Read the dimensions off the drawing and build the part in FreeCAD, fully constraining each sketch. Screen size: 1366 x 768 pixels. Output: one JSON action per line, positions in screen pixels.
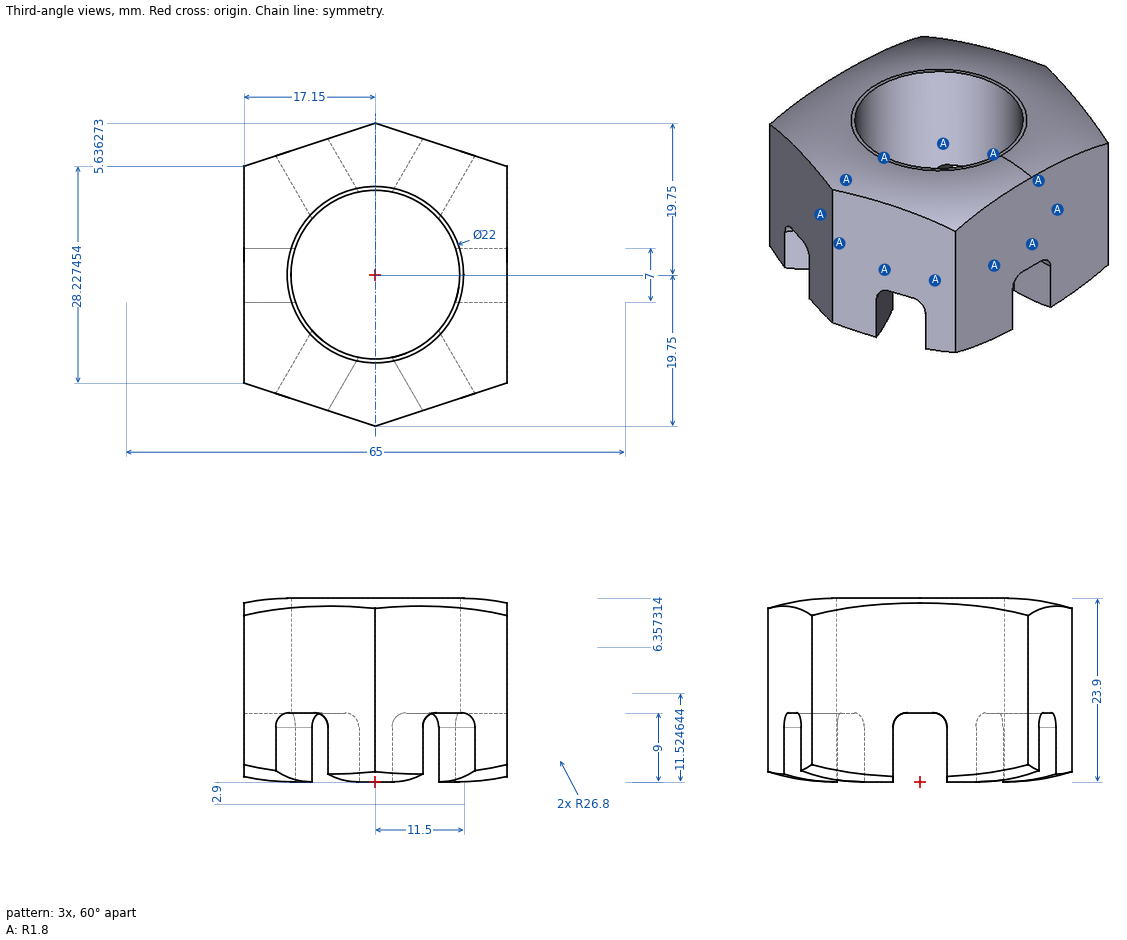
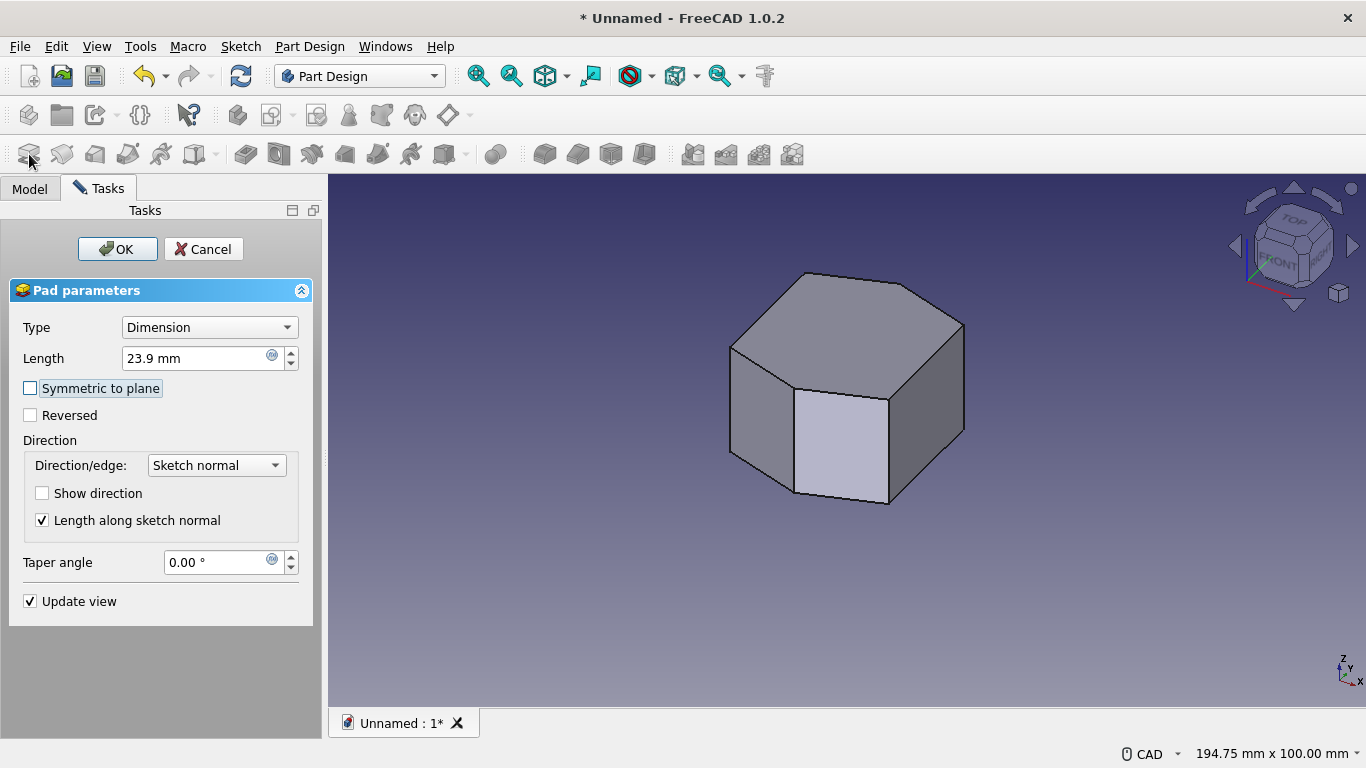
{"action": "left_click", "coordinate": [118, 249]}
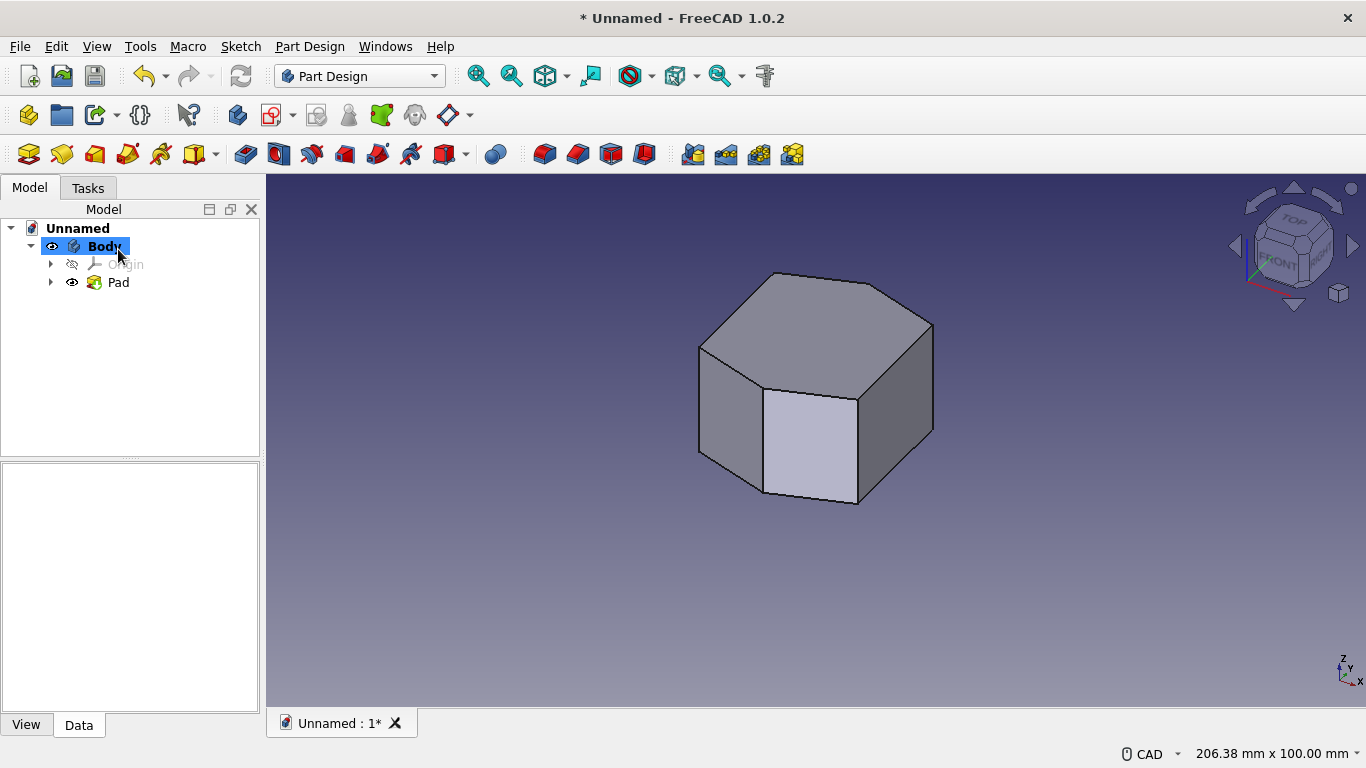
{"action": "left_click", "coordinate": [270, 116]}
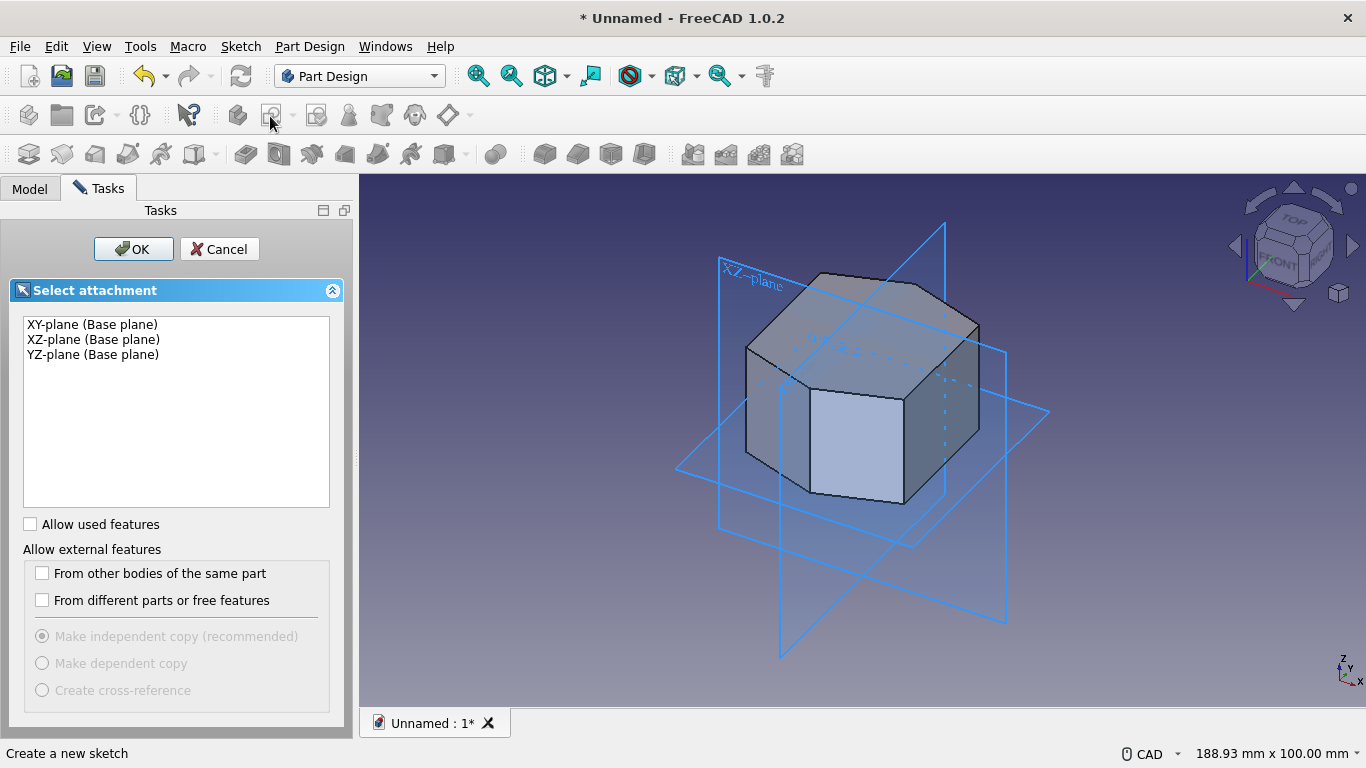
{"action": "left_click", "coordinate": [84, 324]}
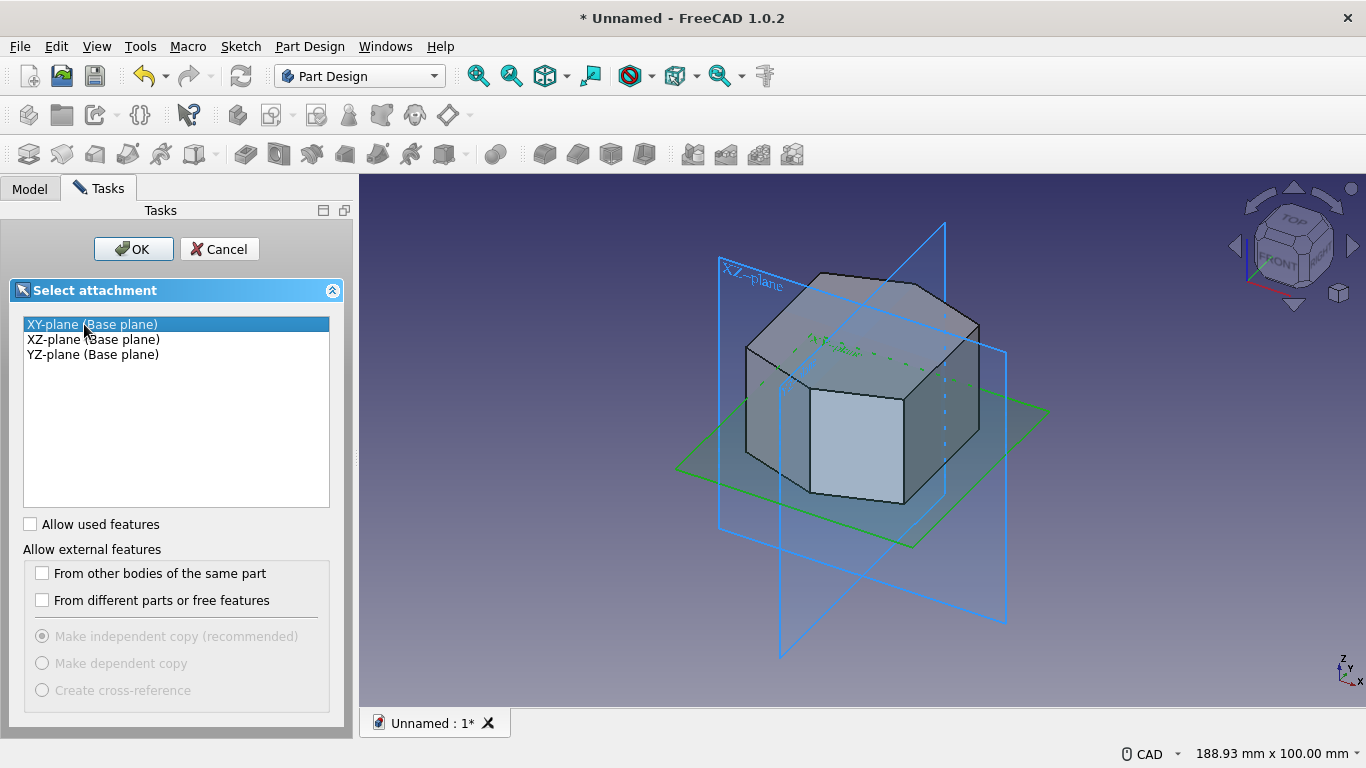
{"action": "left_click", "coordinate": [134, 249]}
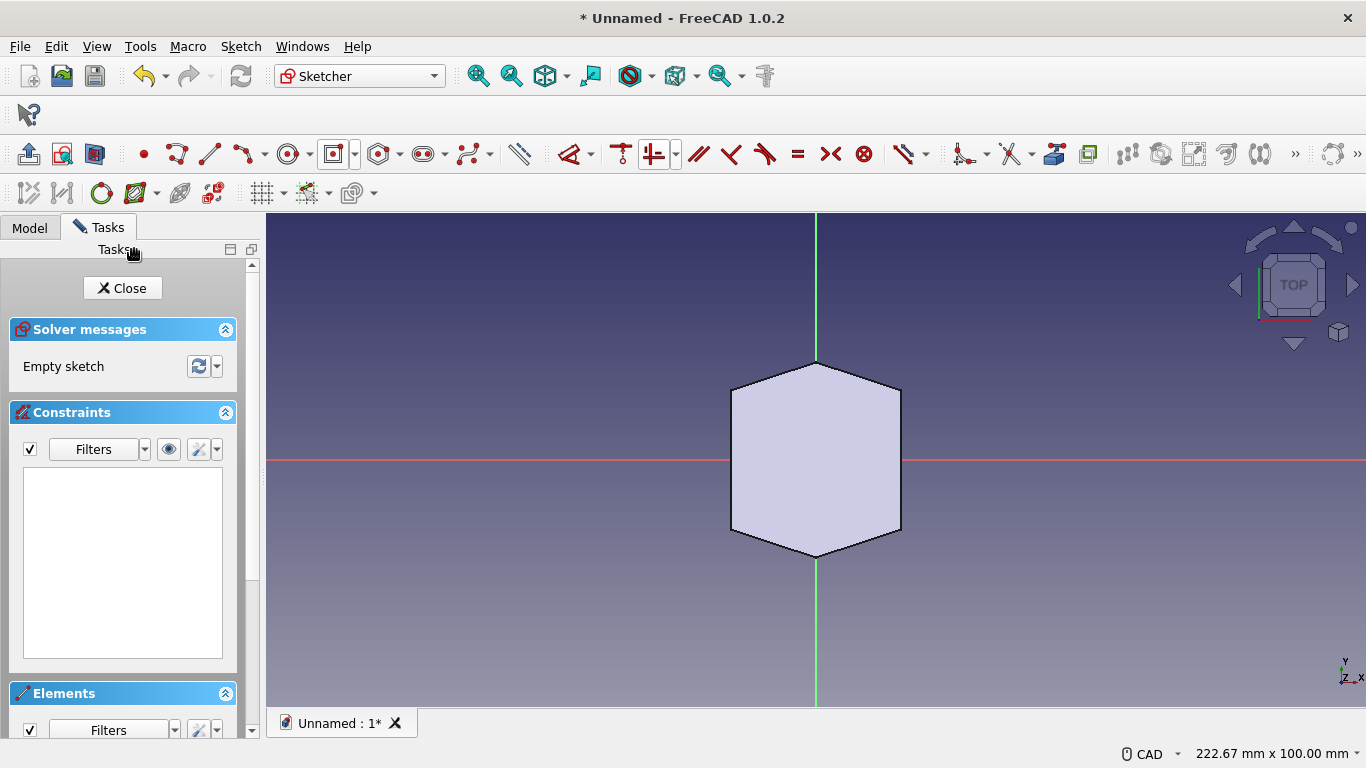
{"action": "left_click", "coordinate": [95, 154]}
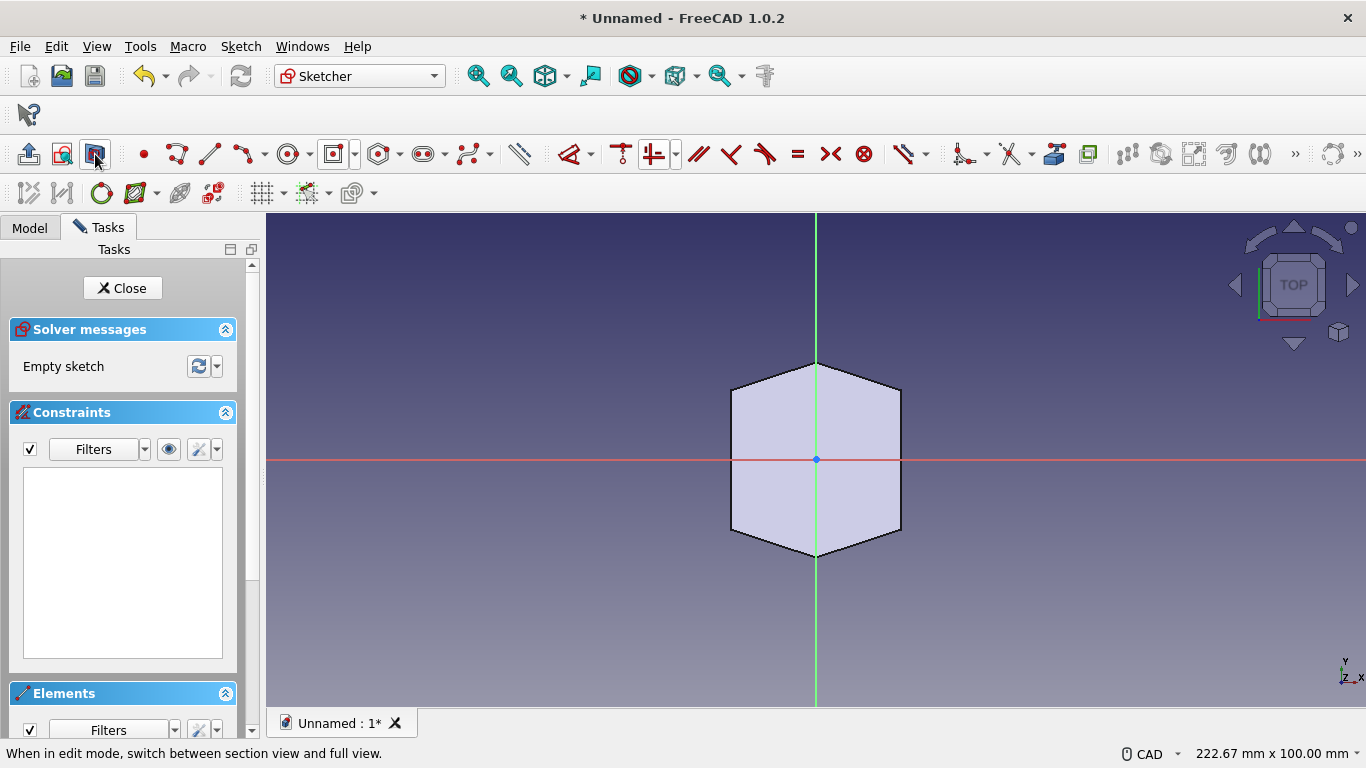
{"action": "scroll", "coordinate": [899, 460], "scroll_direction": "up", "scroll_amount": 3}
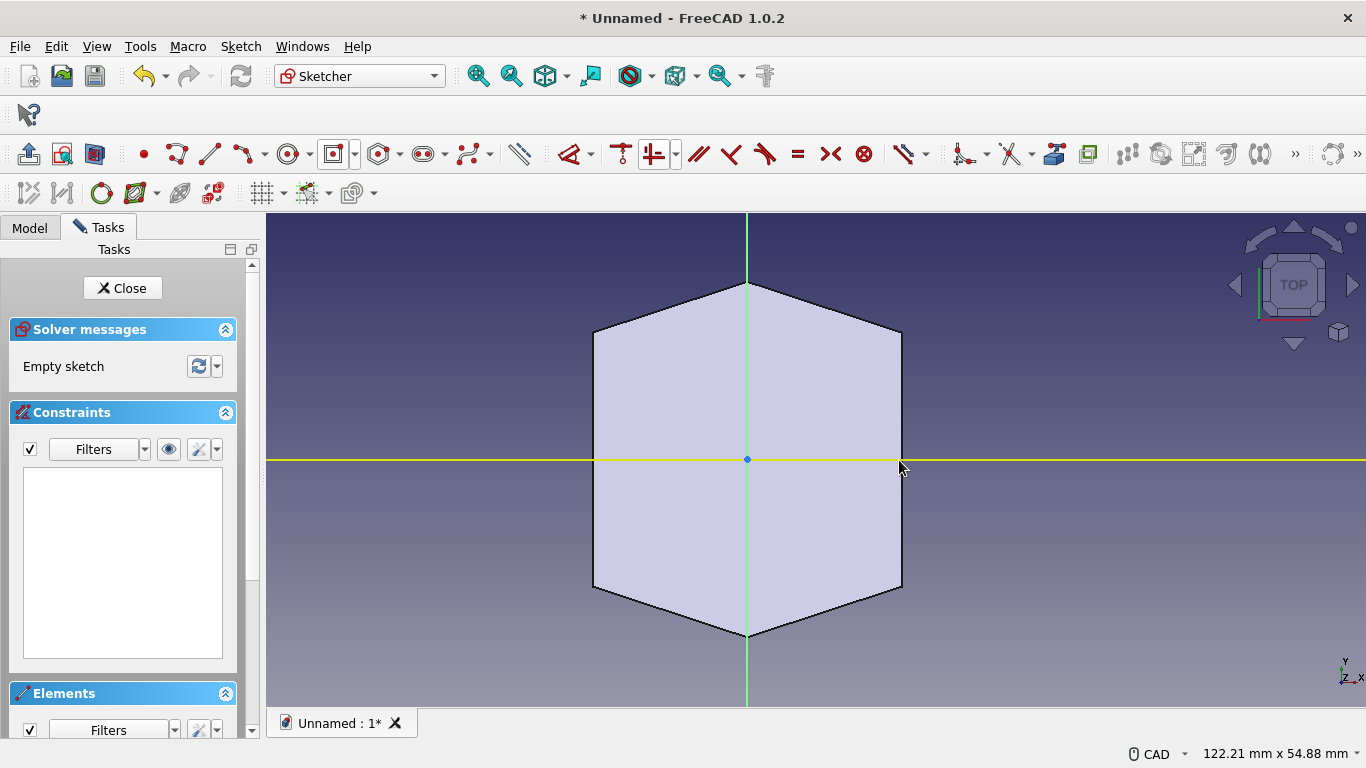
{"action": "left_click", "coordinate": [332, 154]}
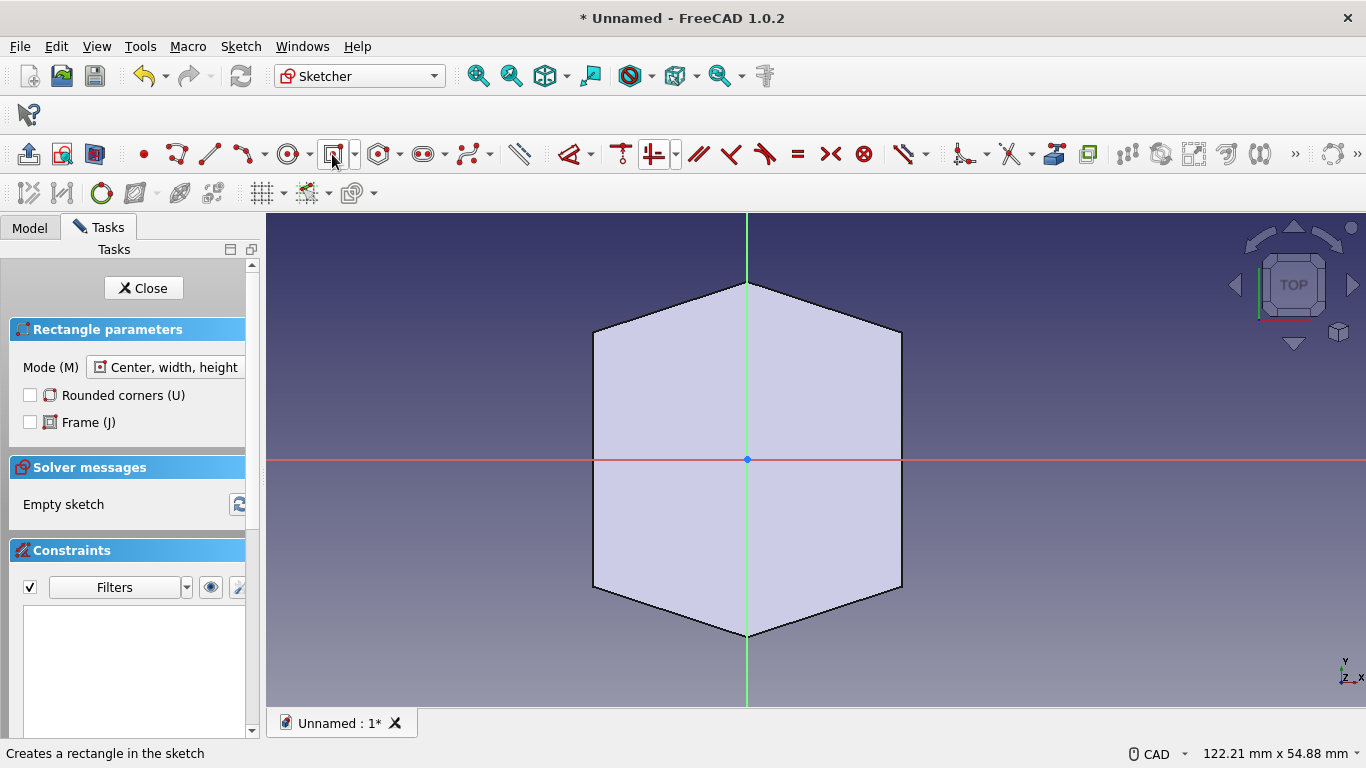
{"action": "left_click", "coordinate": [747, 460]}
{"action": "mouse_move", "coordinate": [1040, 428]}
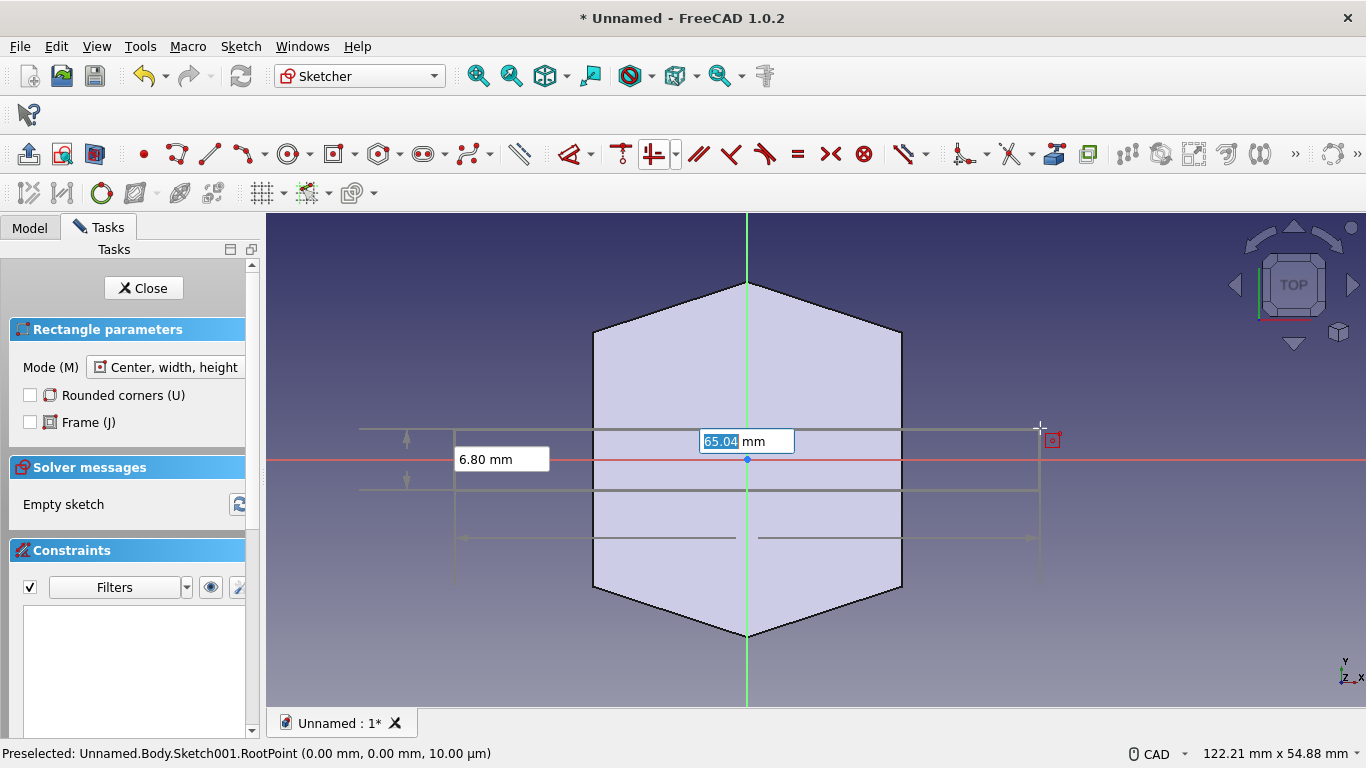
{"action": "type", "text": "65"}
{"action": "key", "text": "Tab"}
{"action": "type", "text": "7"}
{"action": "key", "text": "Return"}
{"action": "key", "text": "Escape"}